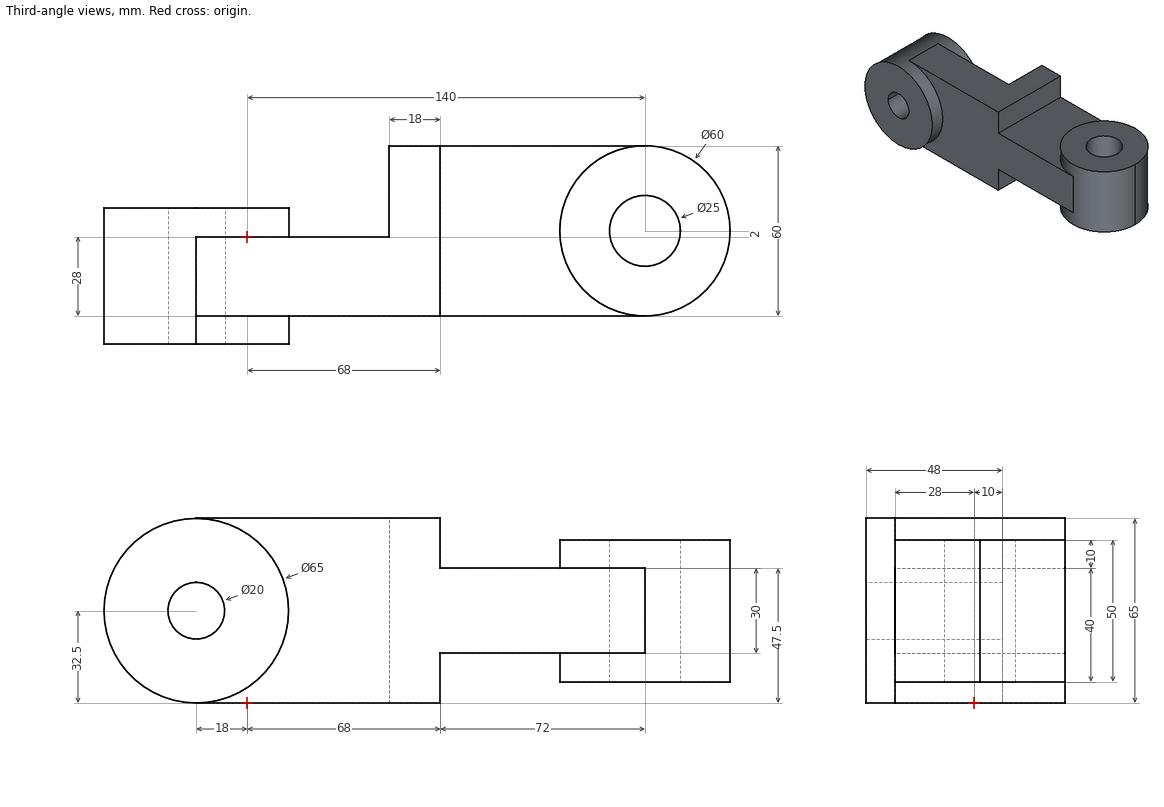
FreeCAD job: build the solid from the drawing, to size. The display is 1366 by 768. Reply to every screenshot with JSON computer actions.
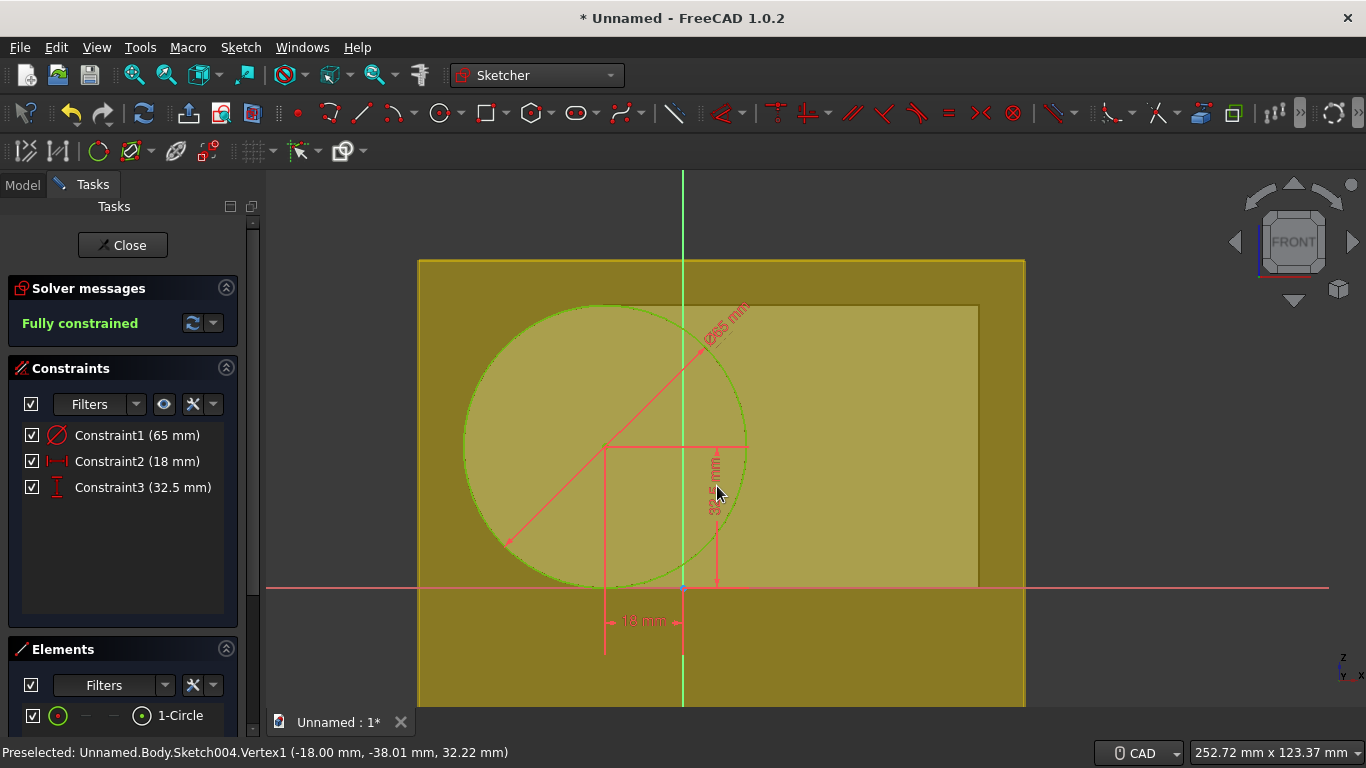
{"action": "left_click", "coordinate": [123, 245]}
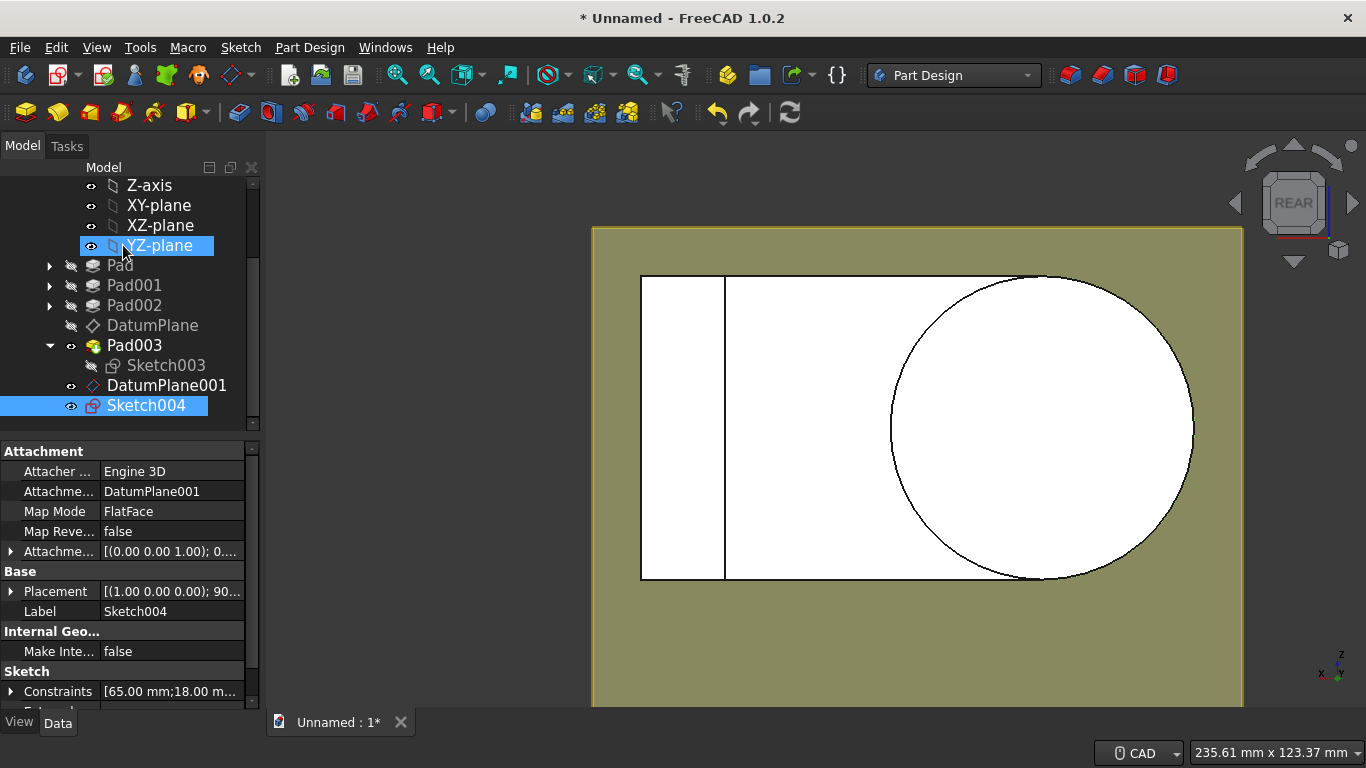
{"action": "left_click", "coordinate": [240, 112]}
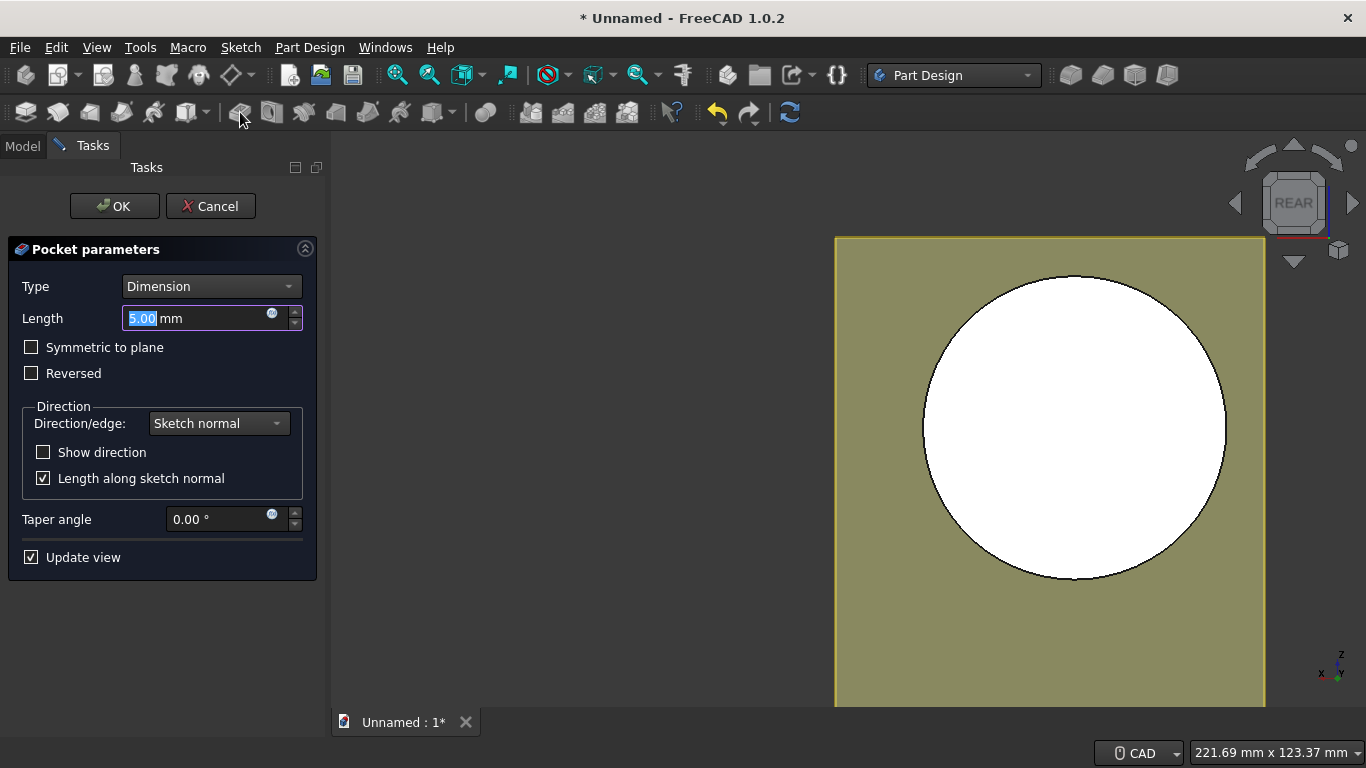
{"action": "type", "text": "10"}
{"action": "key", "text": "Tab"}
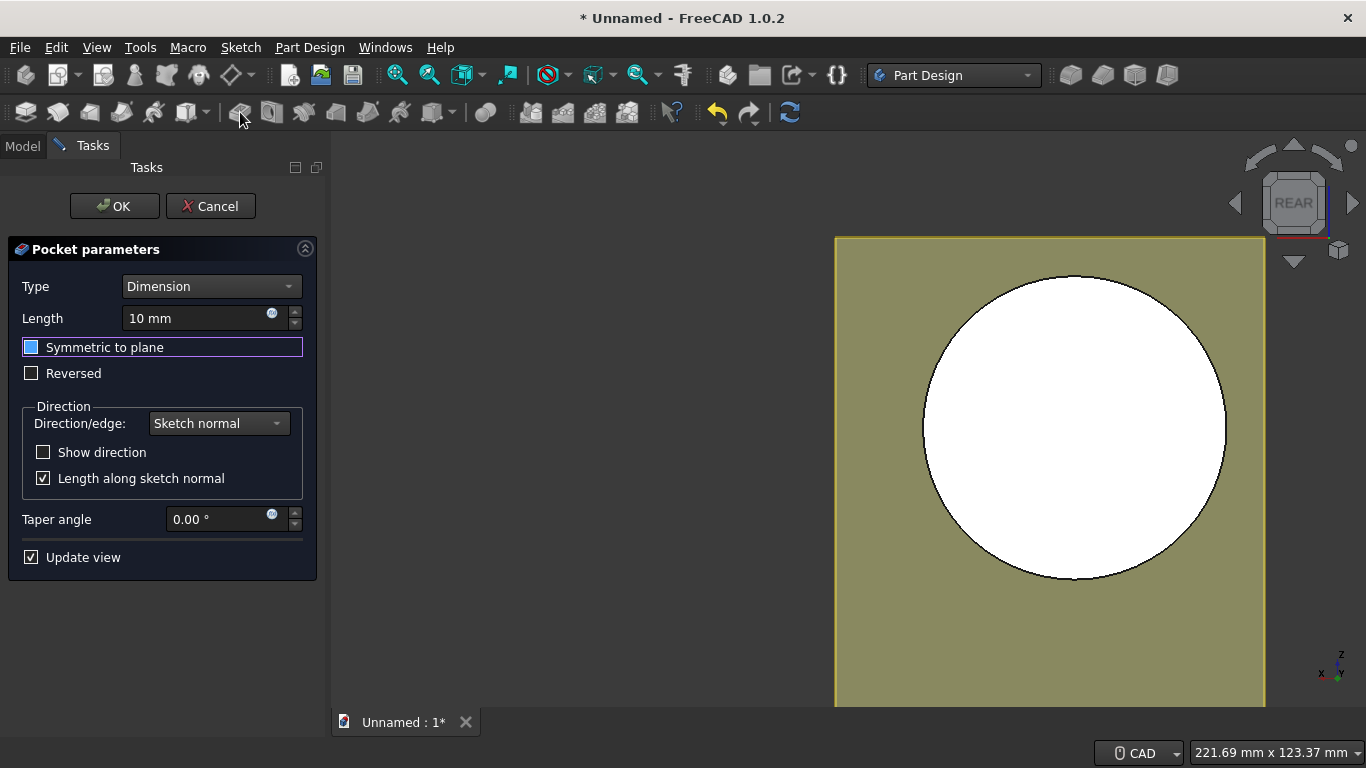
{"action": "left_click", "coordinate": [30, 373]}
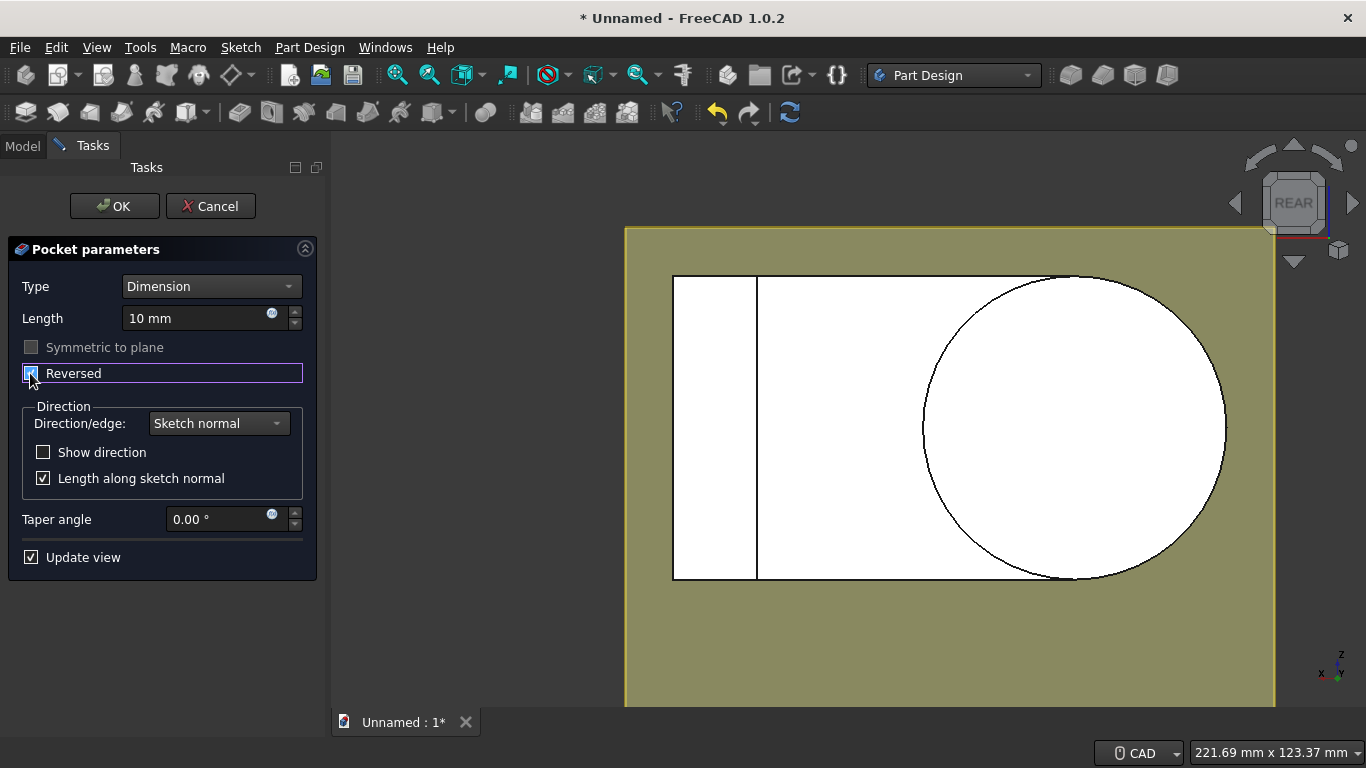
{"action": "left_click", "coordinate": [115, 206]}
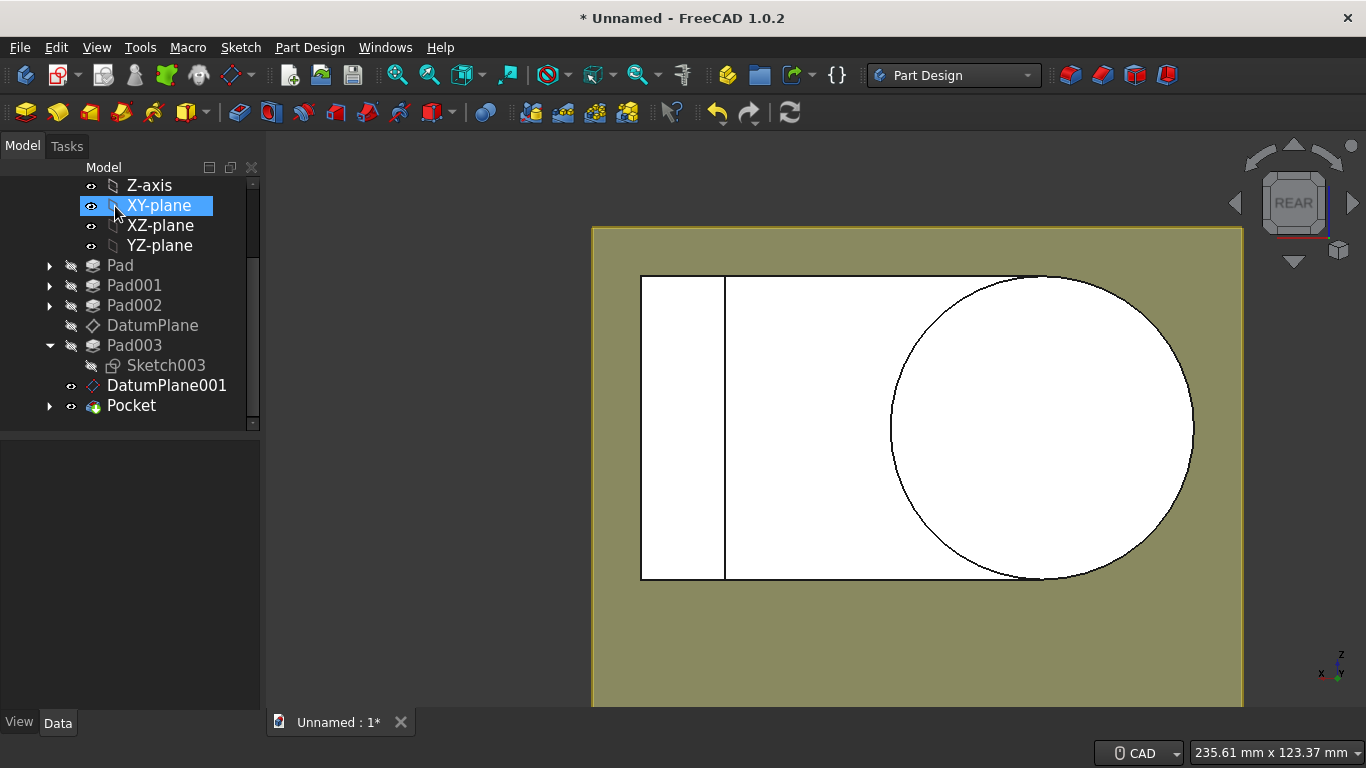
{"action": "left_click", "coordinate": [116, 386]}
{"action": "key", "text": "space"}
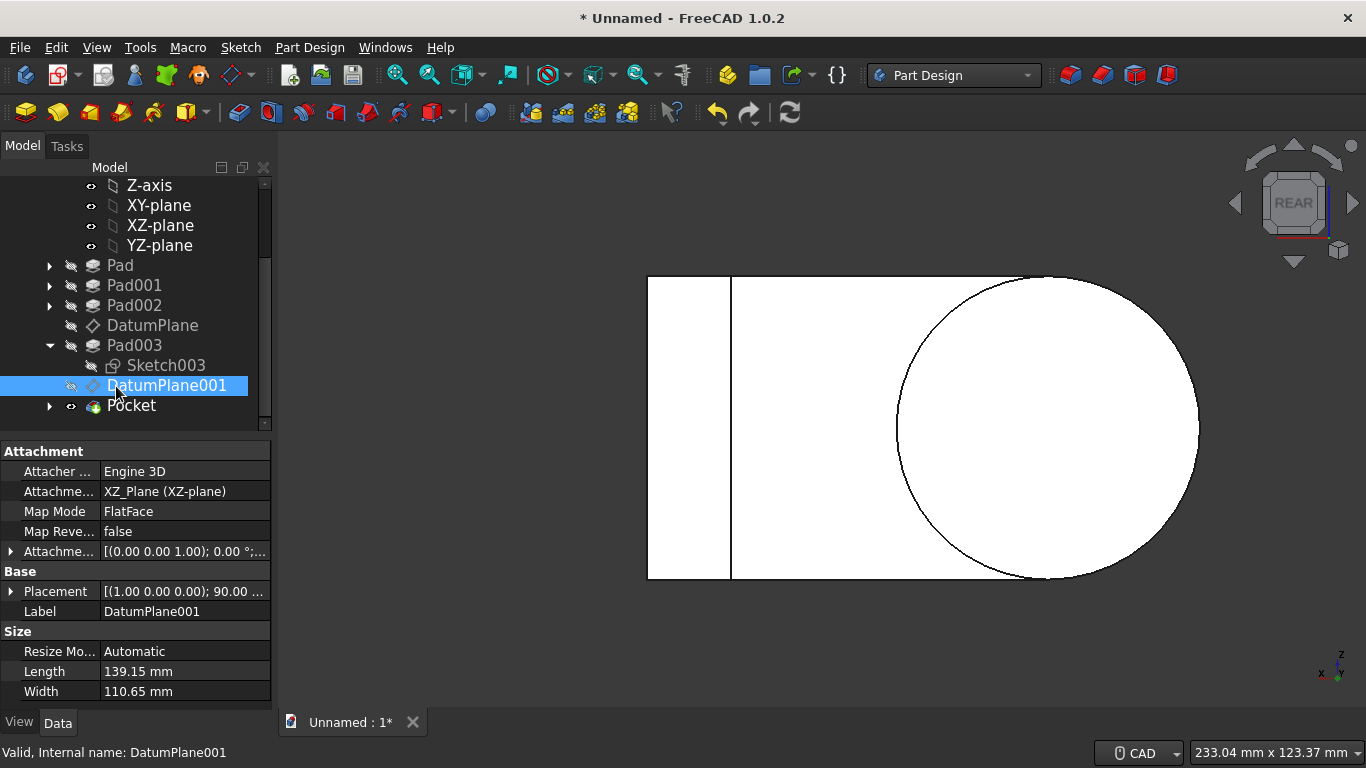
{"action": "left_click", "coordinate": [1048, 427]}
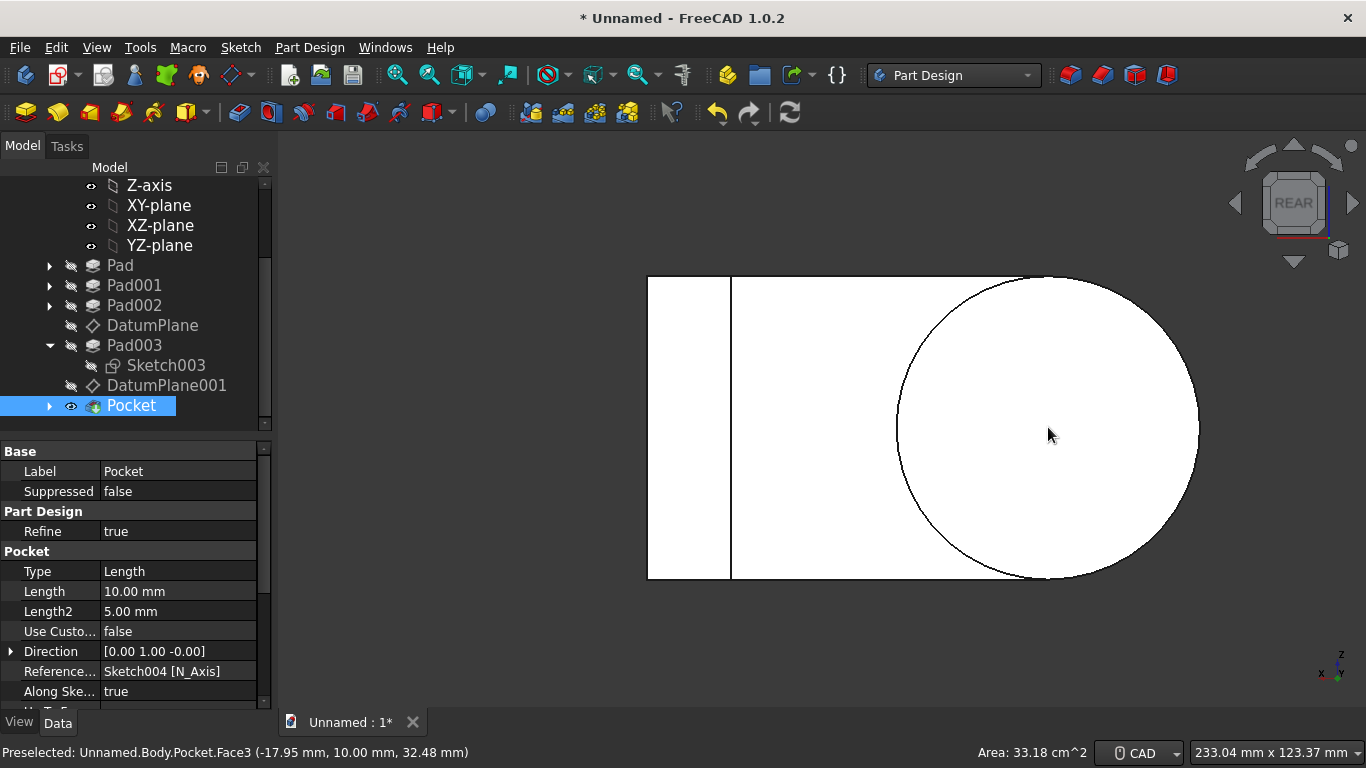
{"action": "left_click", "coordinate": [58, 76]}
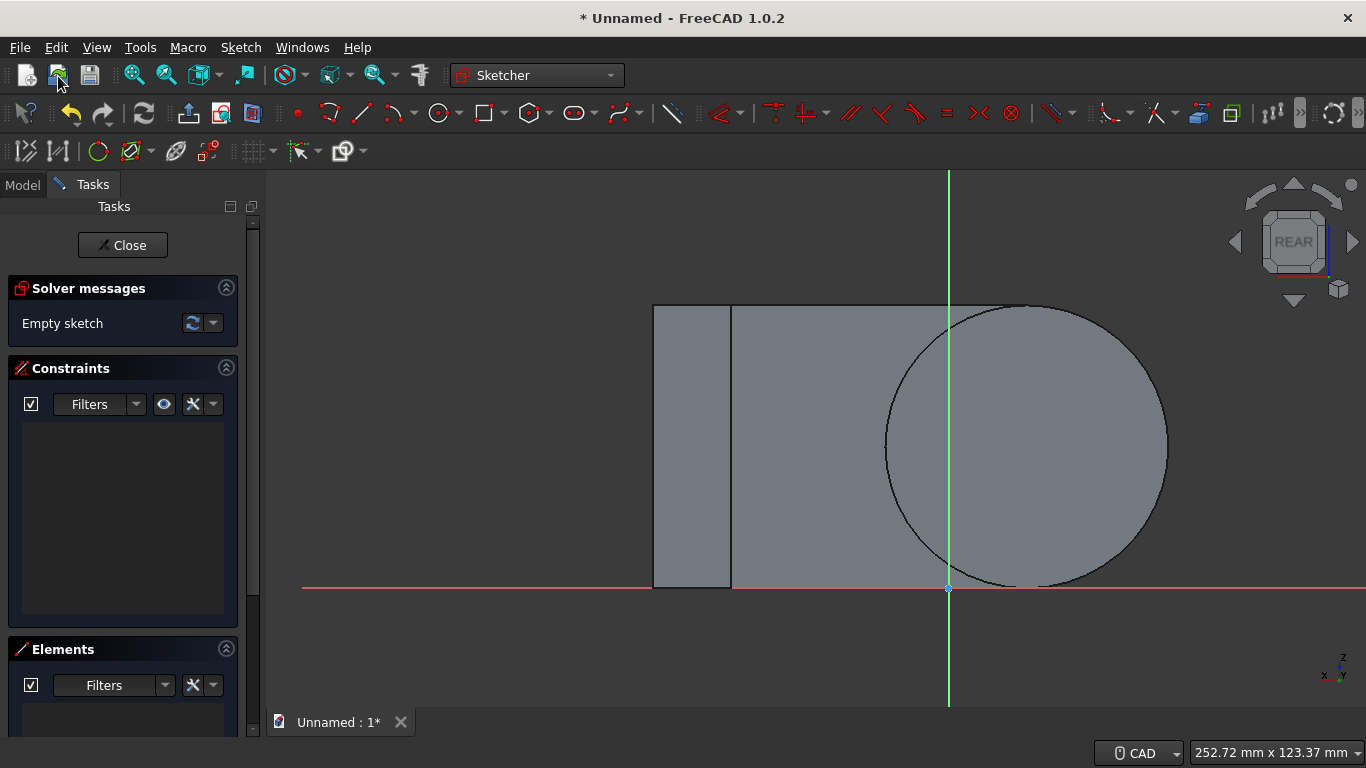
{"action": "key", "text": "q s"}